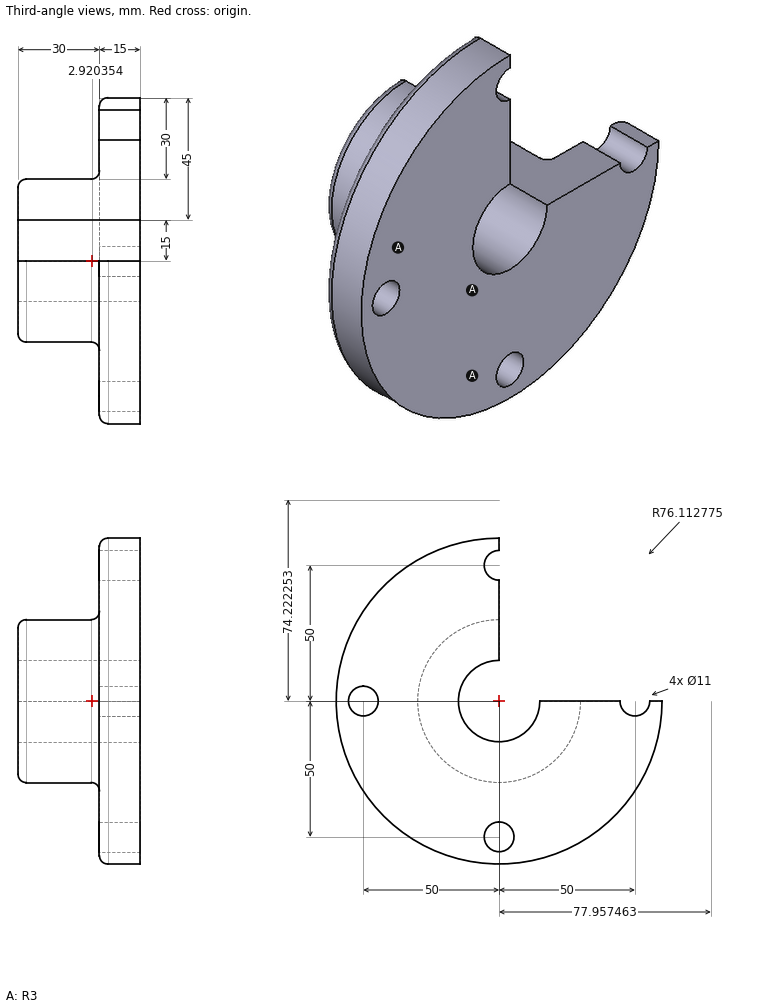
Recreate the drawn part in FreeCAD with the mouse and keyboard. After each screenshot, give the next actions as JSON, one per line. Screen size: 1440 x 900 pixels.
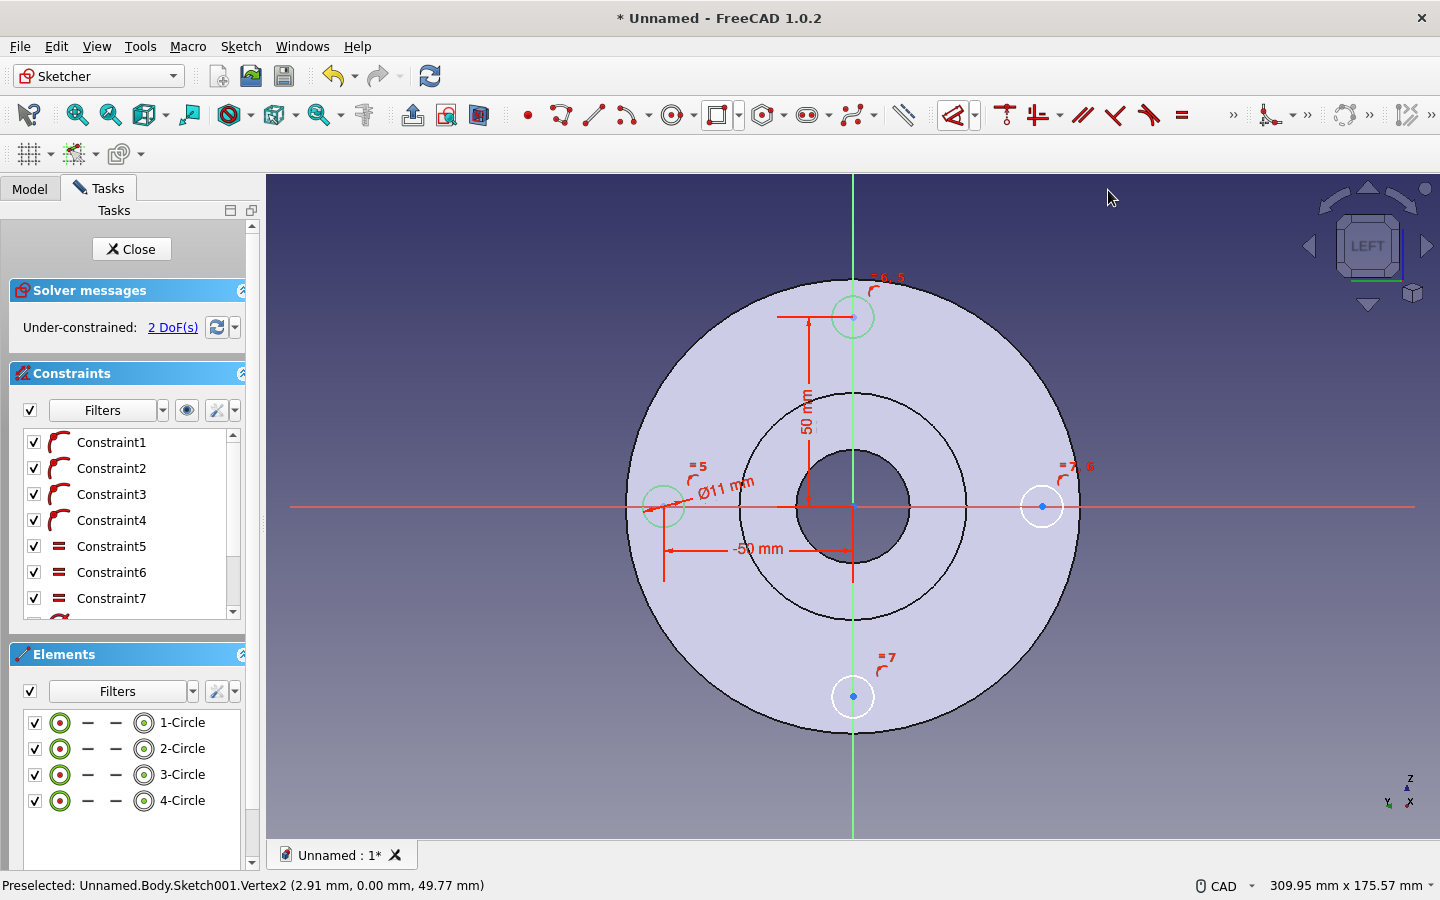
{"action": "left_click", "coordinate": [1042, 506]}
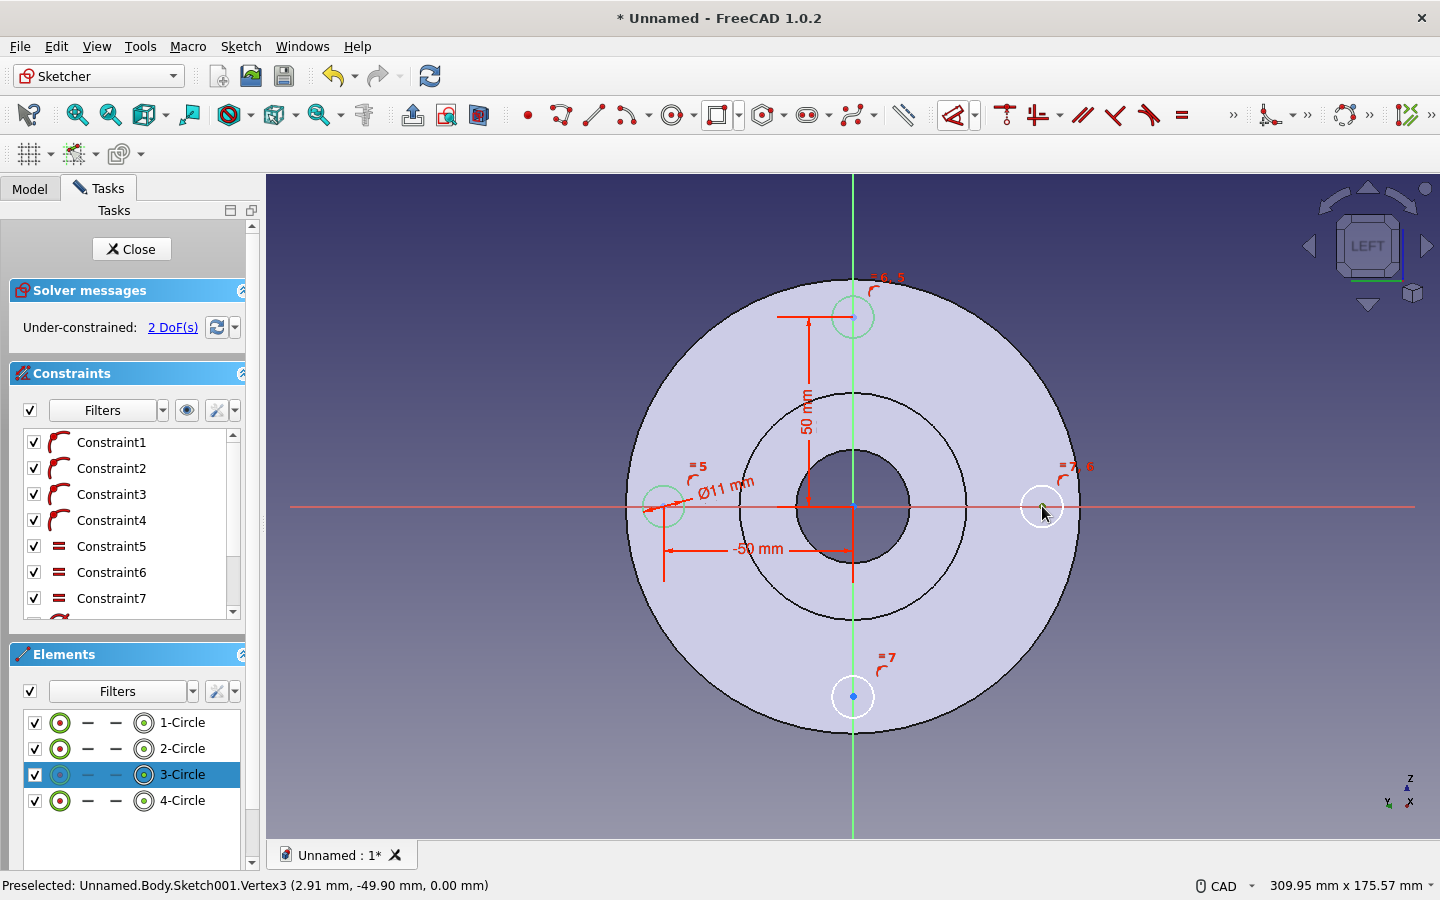
{"action": "left_click", "coordinate": [974, 116]}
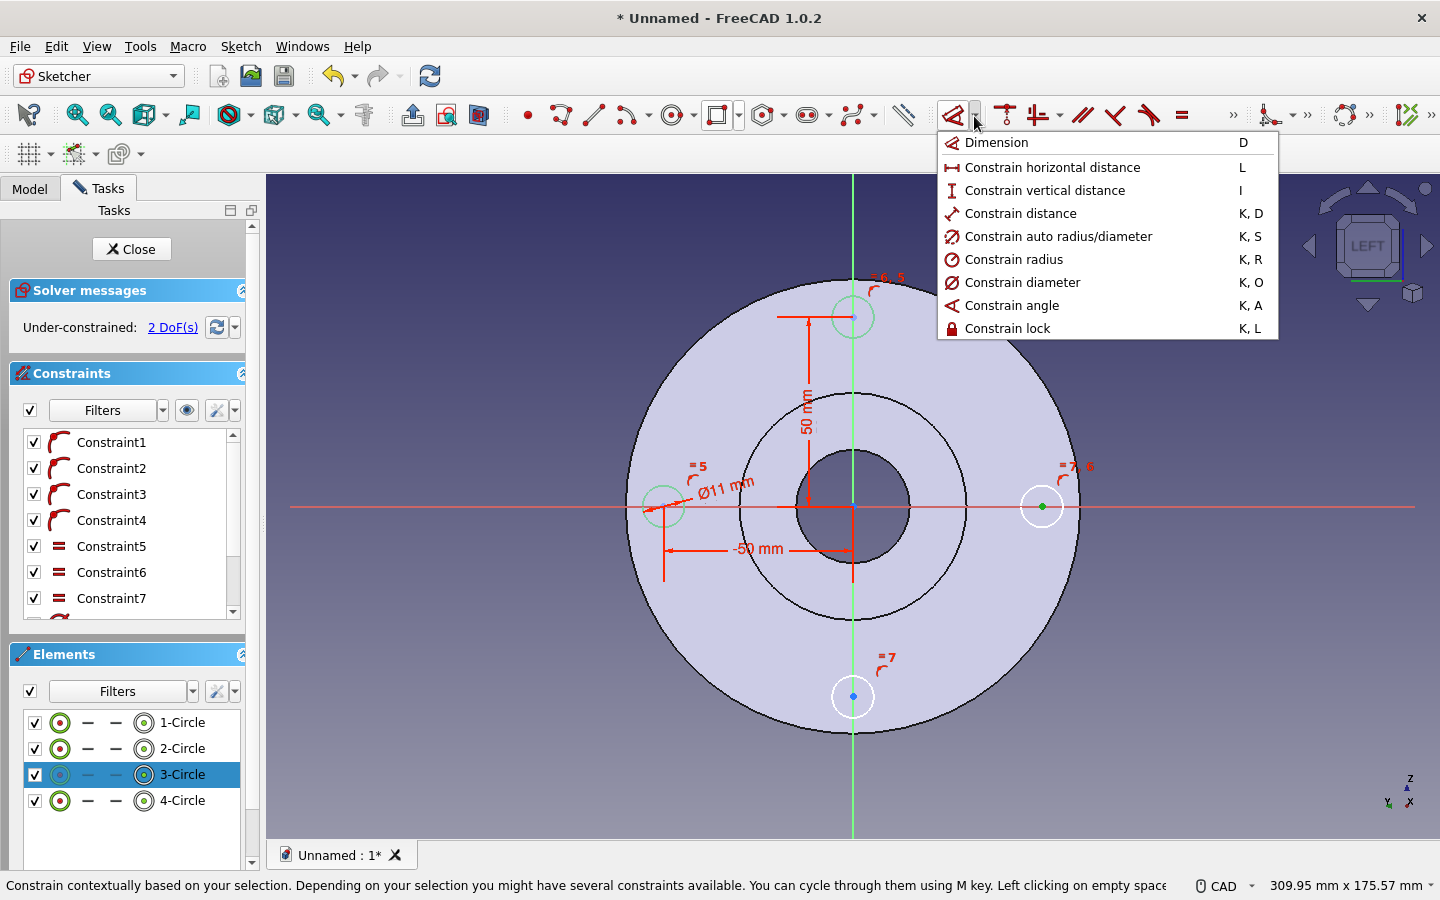
{"action": "left_click", "coordinate": [1108, 168]}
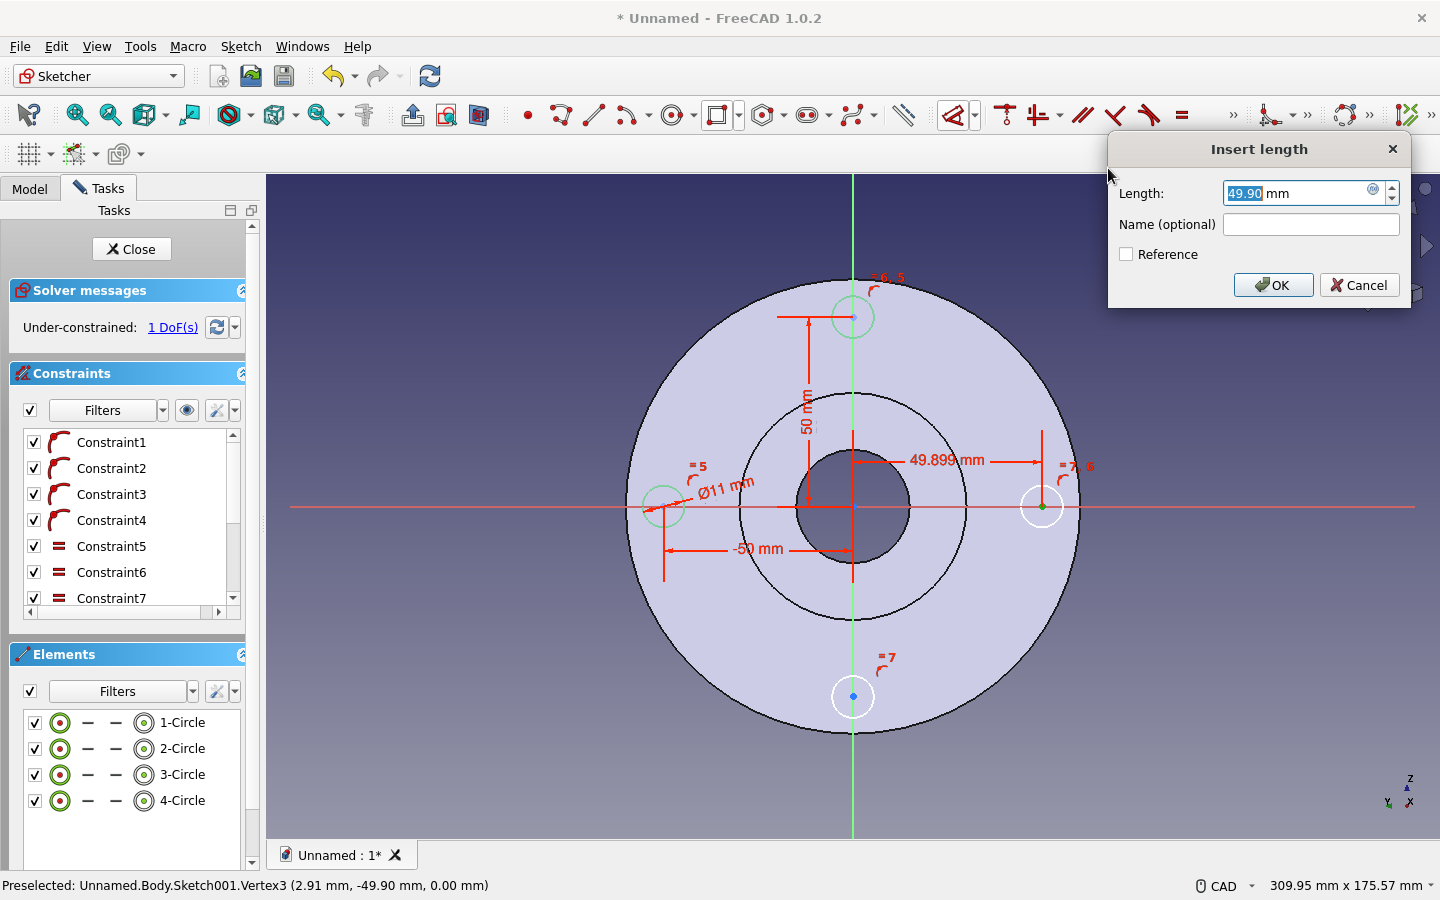
{"action": "type", "text": "50"}
{"action": "key", "text": "Return"}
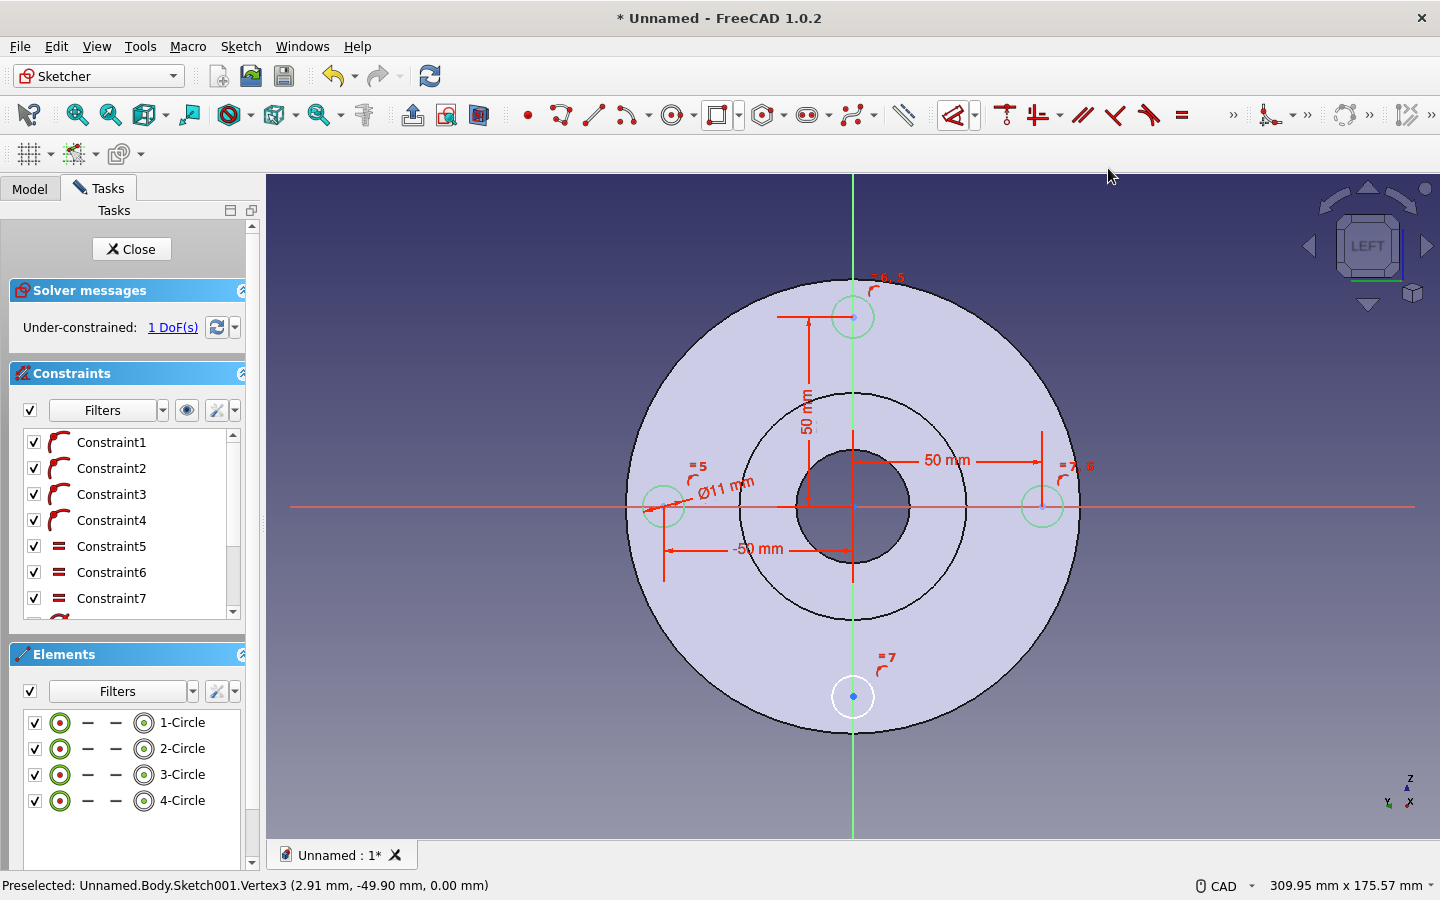
{"action": "left_click", "coordinate": [853, 697]}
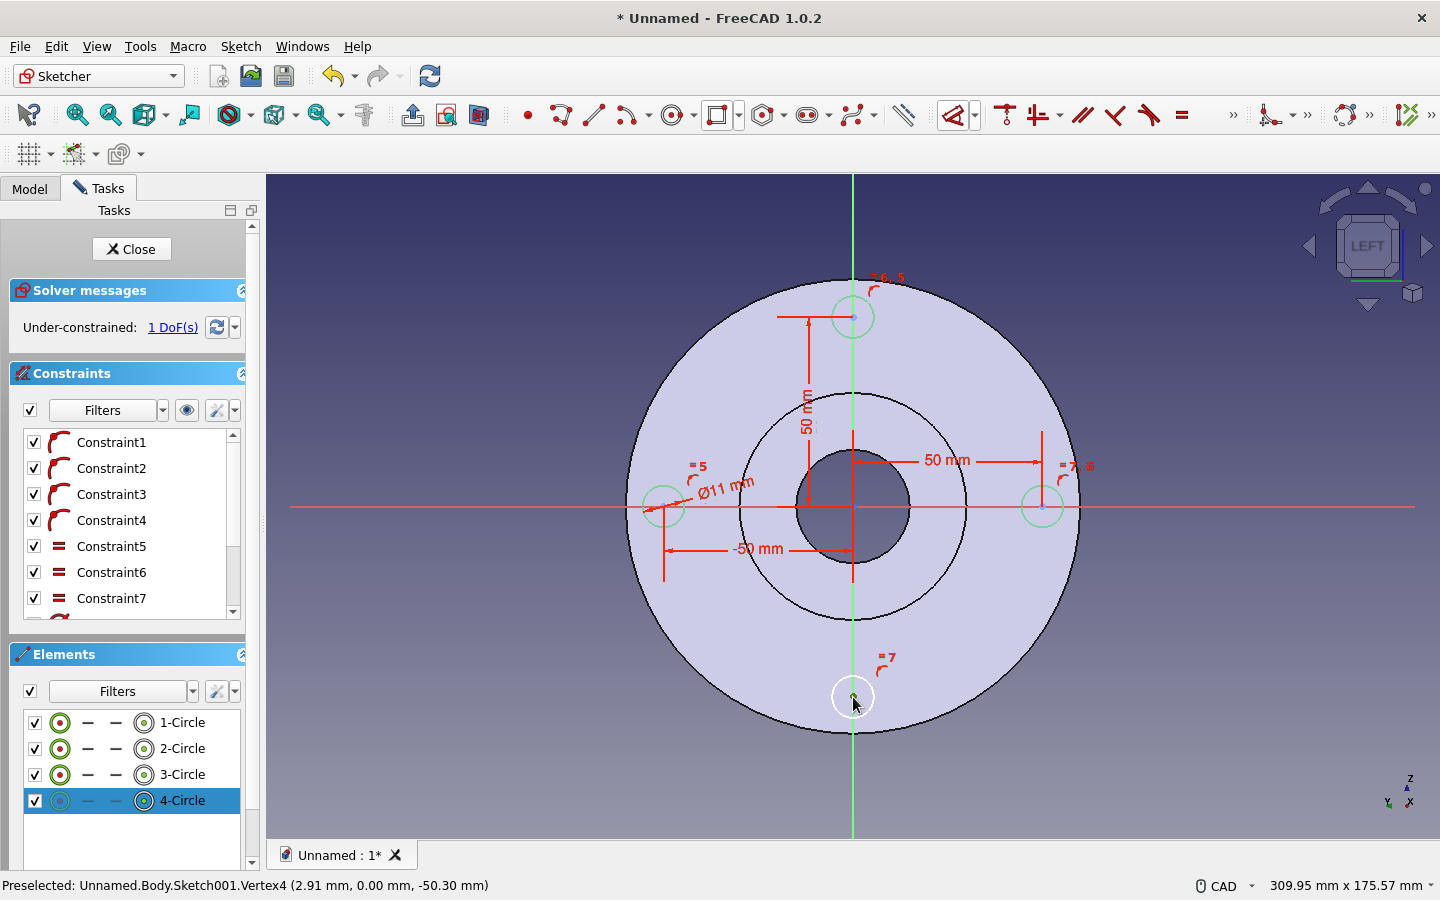
{"action": "left_click", "coordinate": [974, 116]}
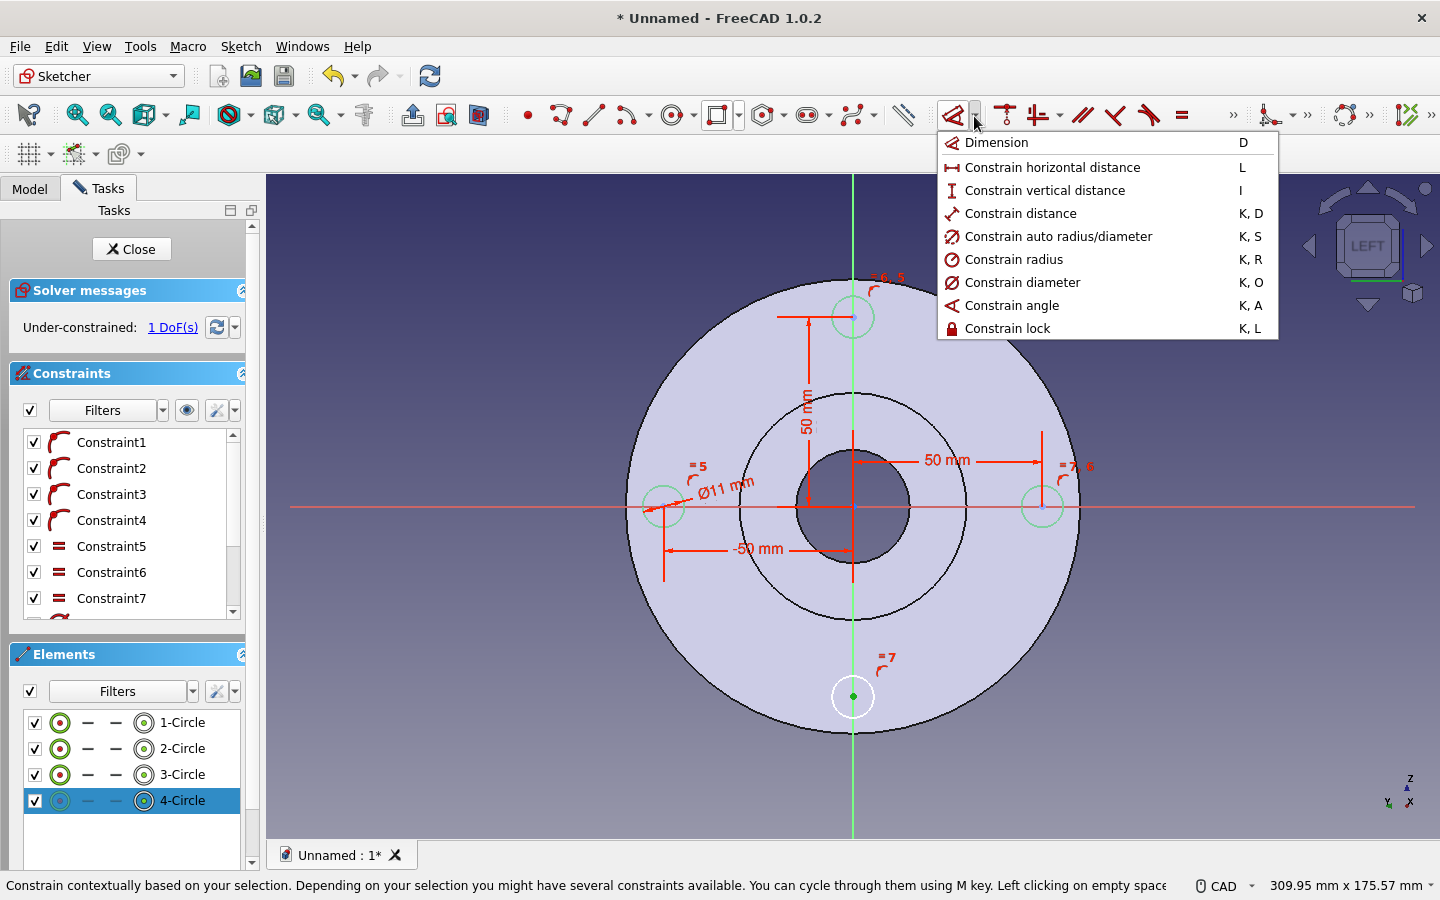
{"action": "left_click", "coordinate": [1108, 190]}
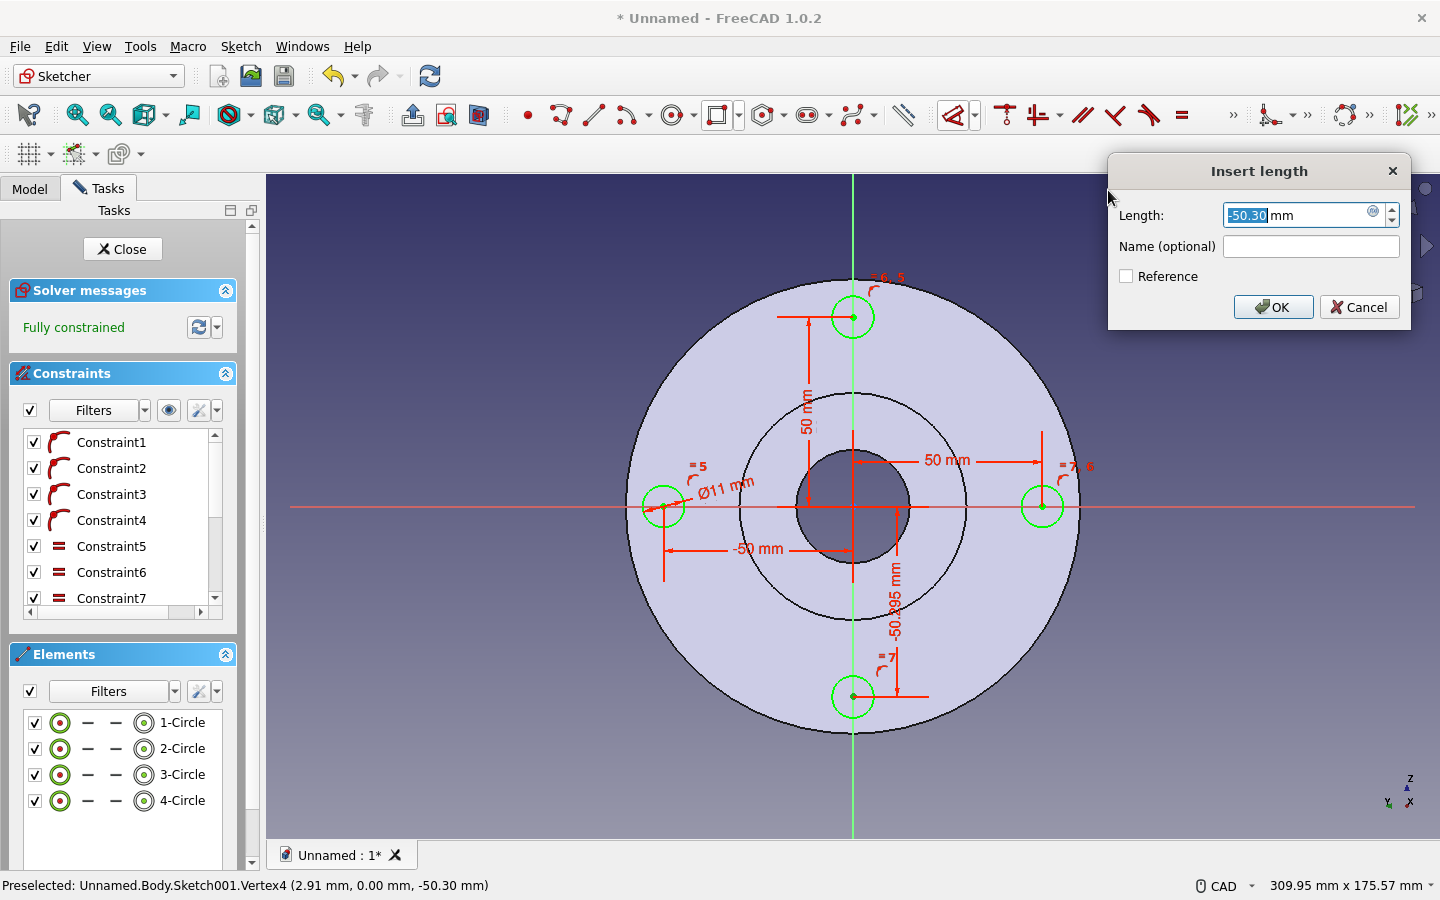
{"action": "type", "text": "-50"}
{"action": "key", "text": "Return"}